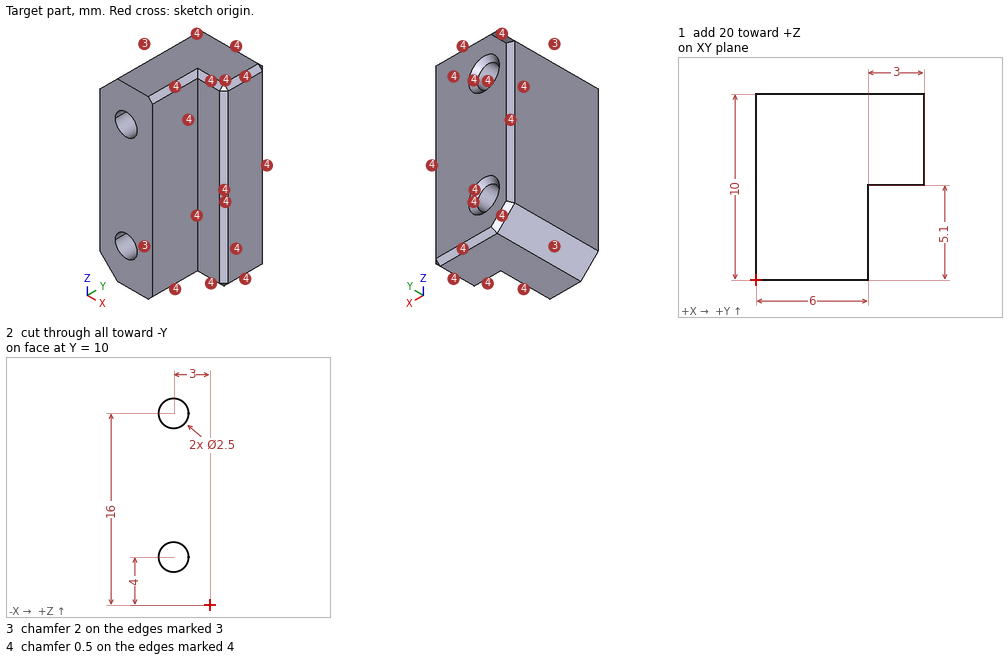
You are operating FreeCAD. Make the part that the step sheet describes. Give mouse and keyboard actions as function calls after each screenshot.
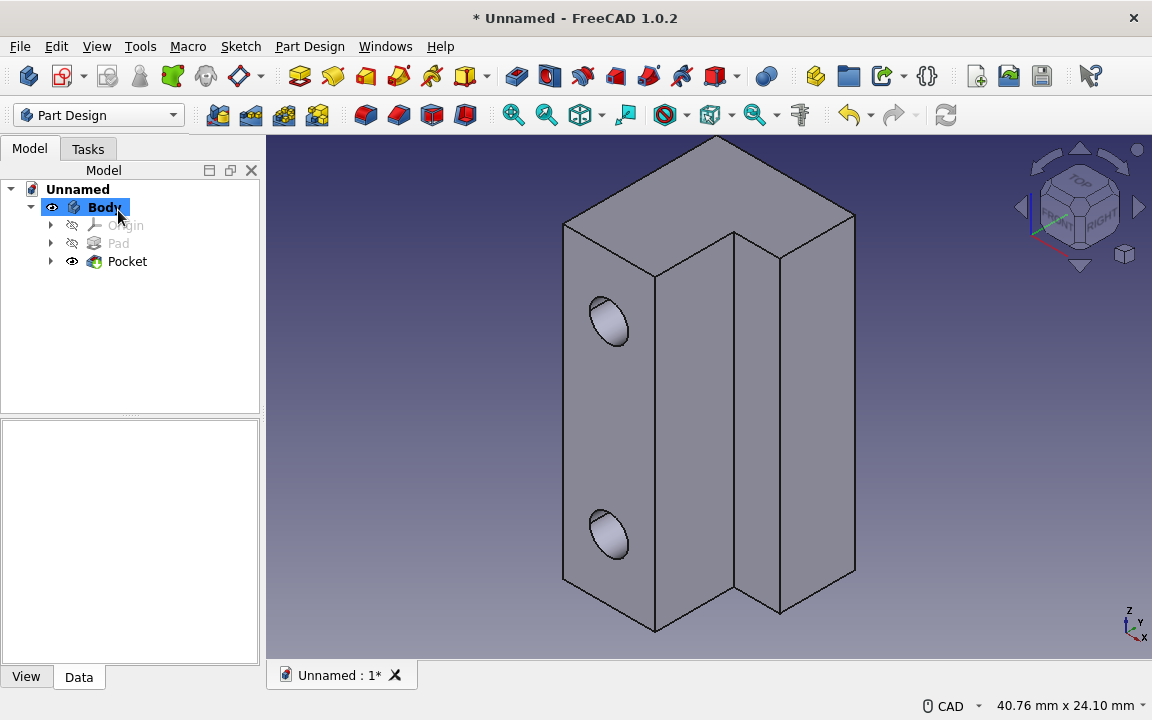
click(514, 116)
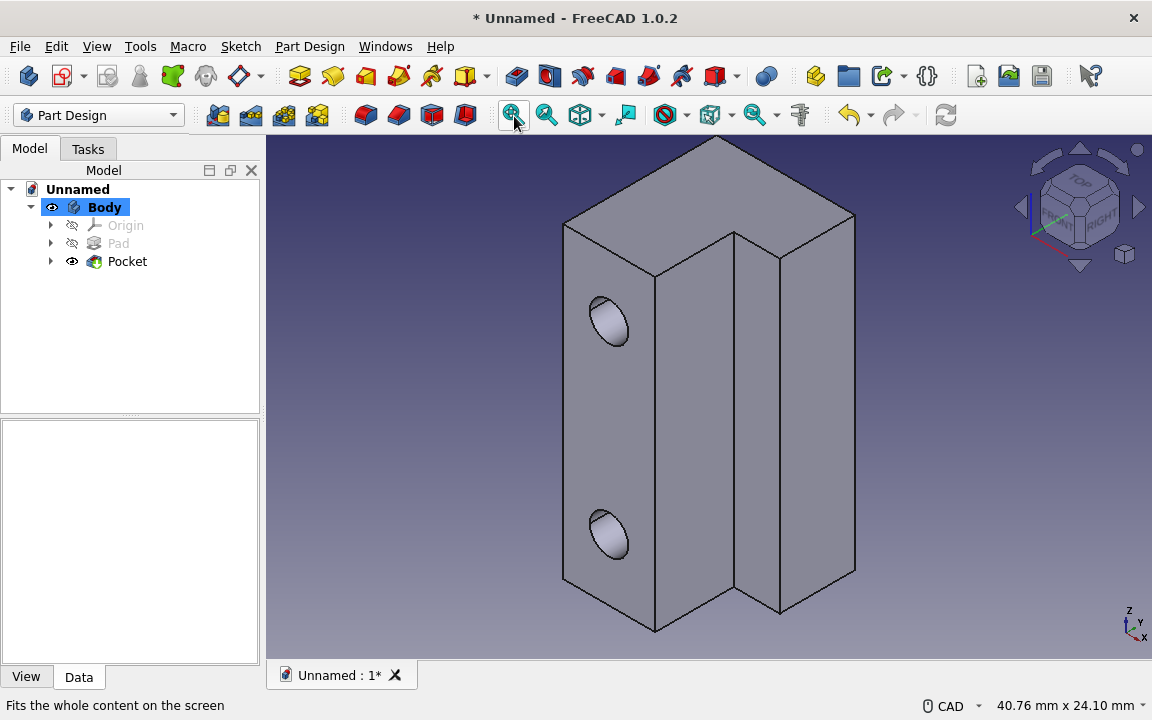
key(2)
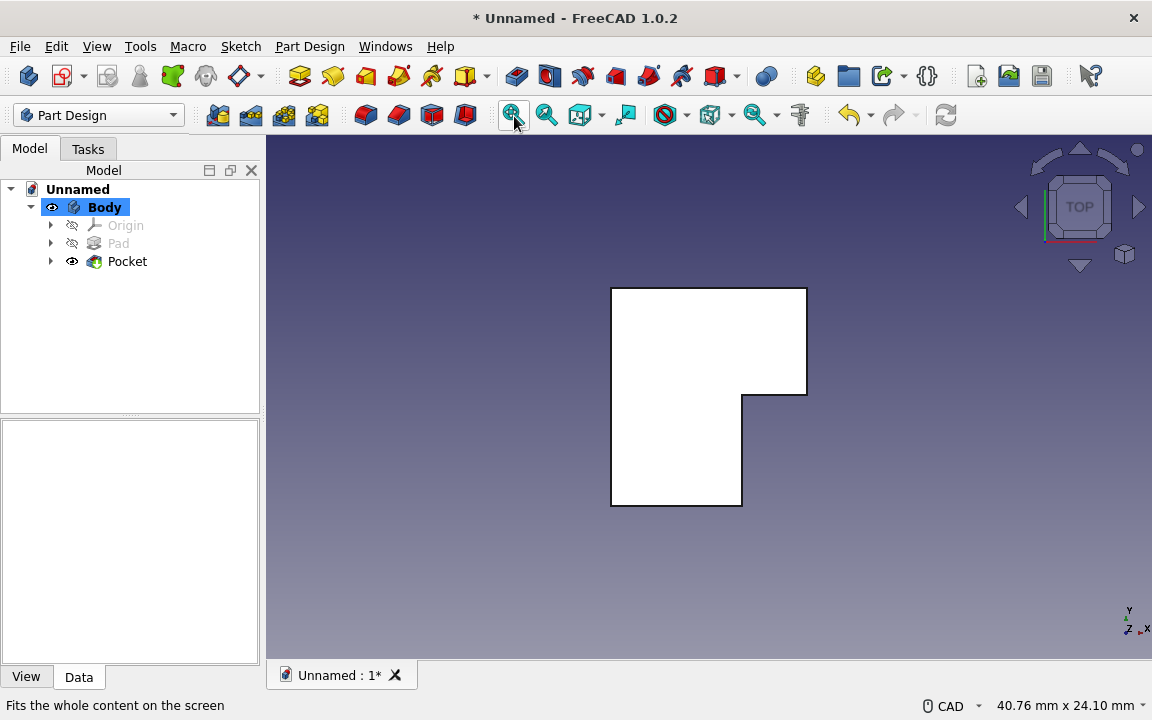
click(514, 116)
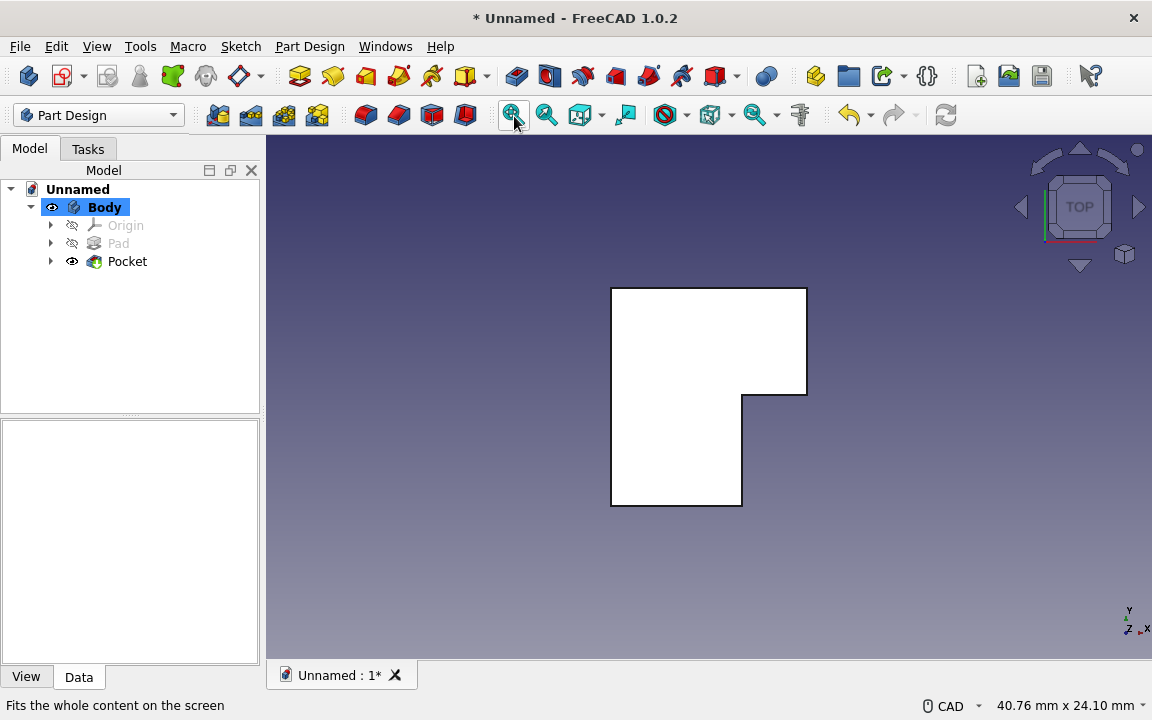
click(611, 396)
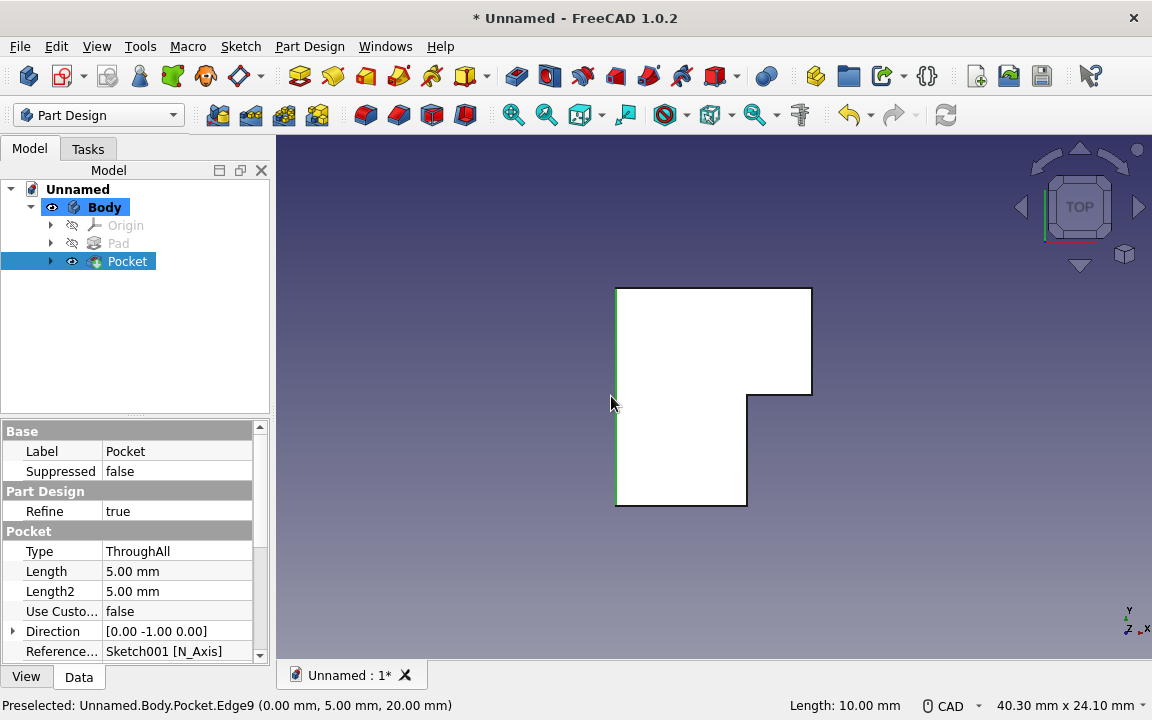
key(1)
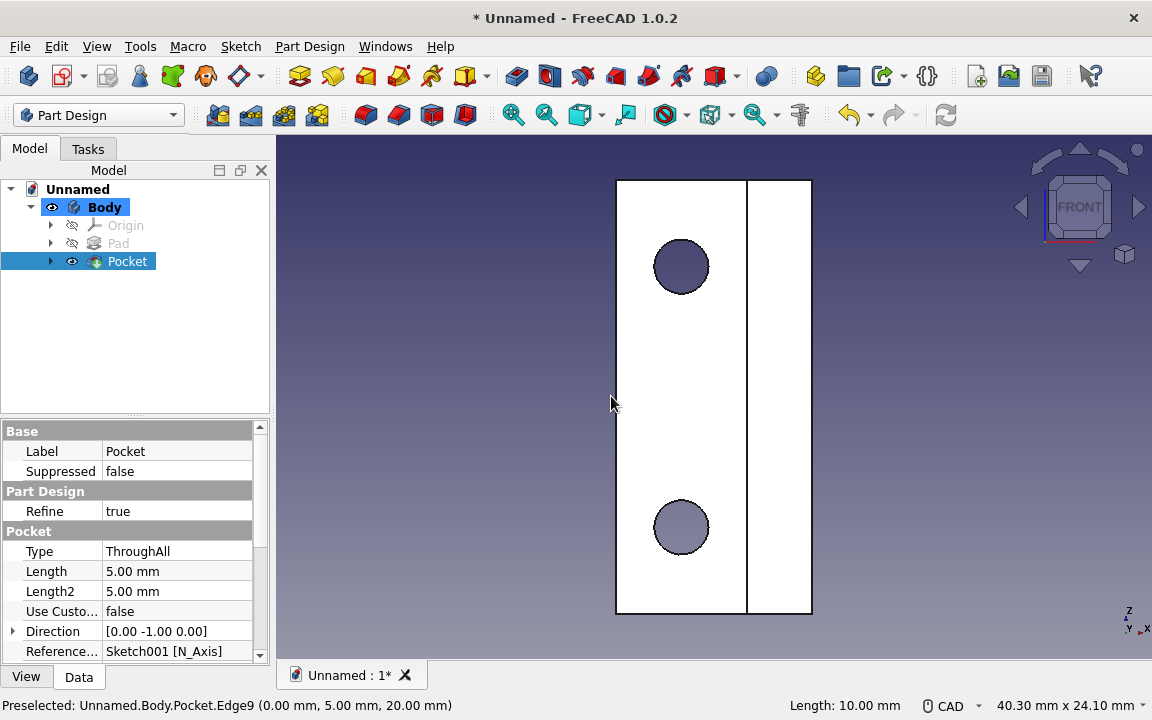
key(3)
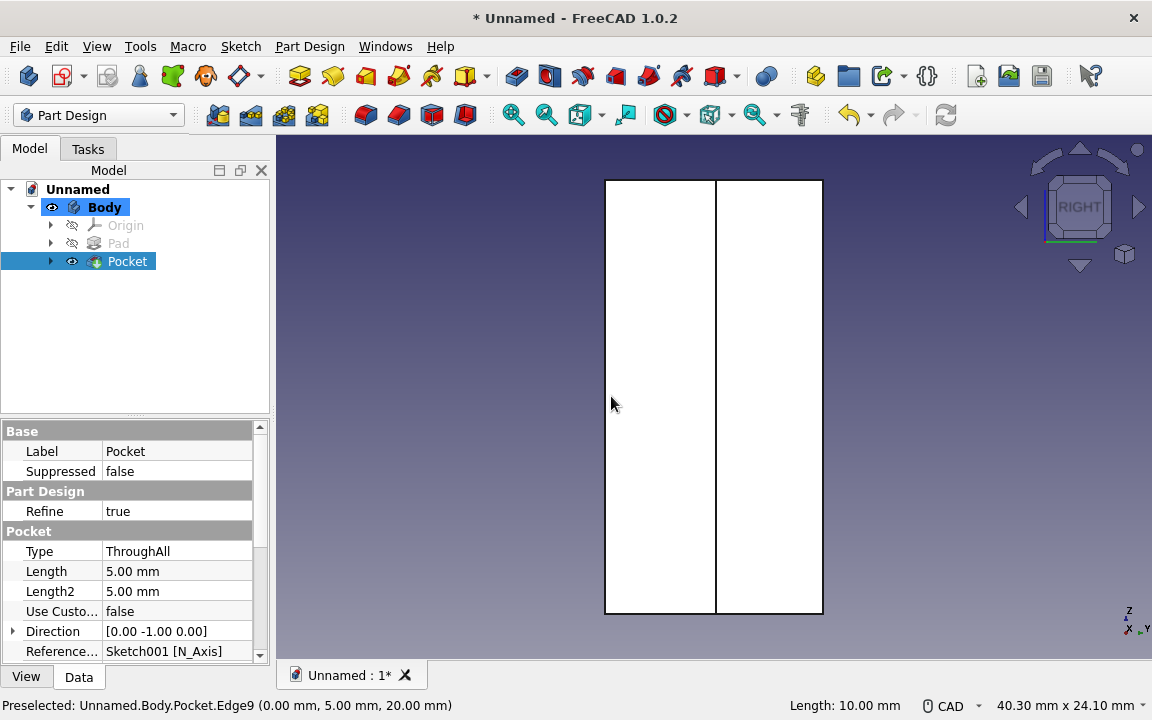
key(5)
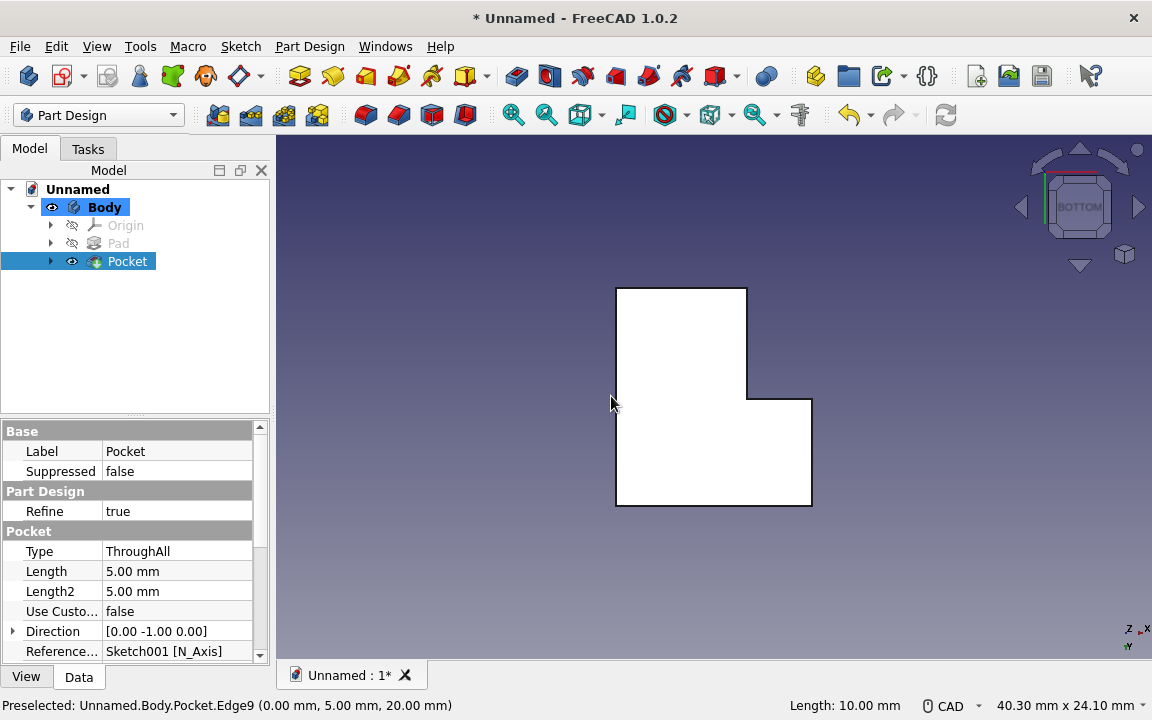
click(514, 116)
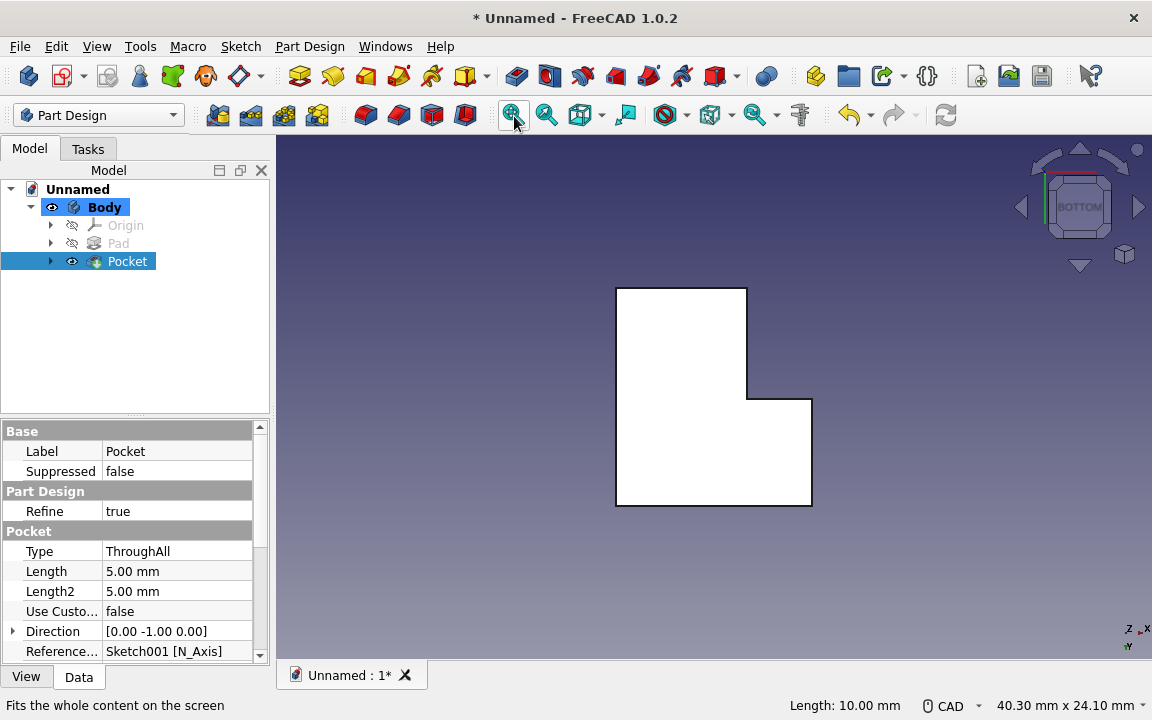
click(616, 396, ctrl)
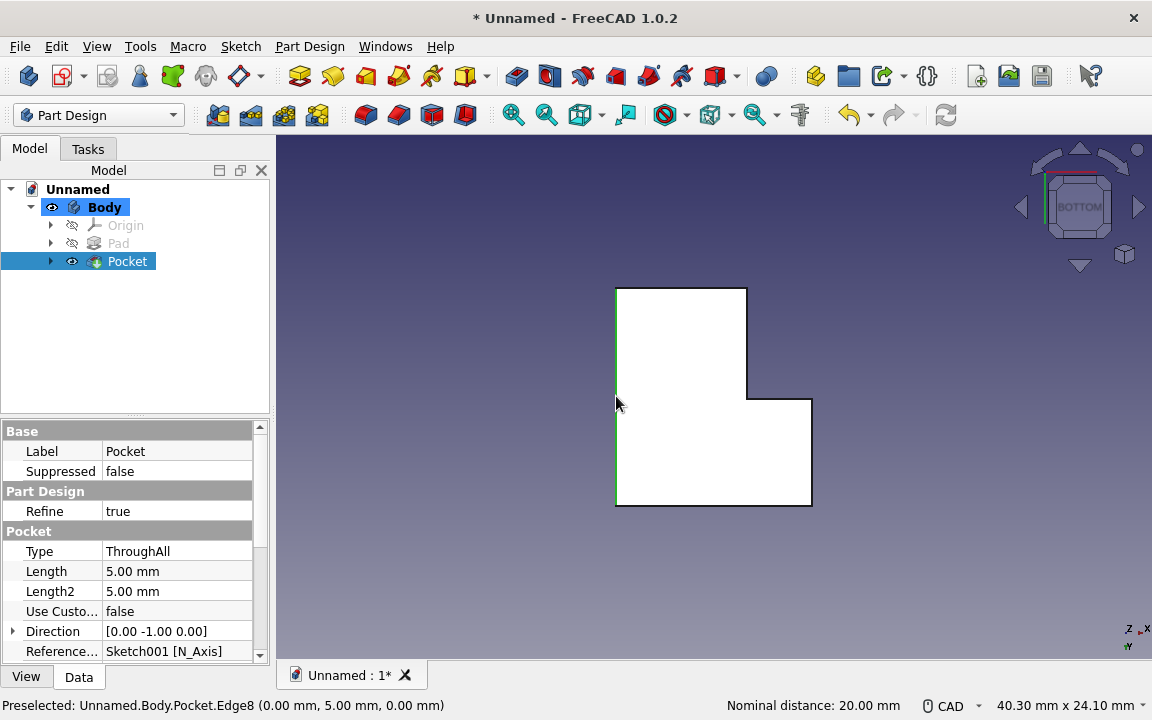
click(399, 116)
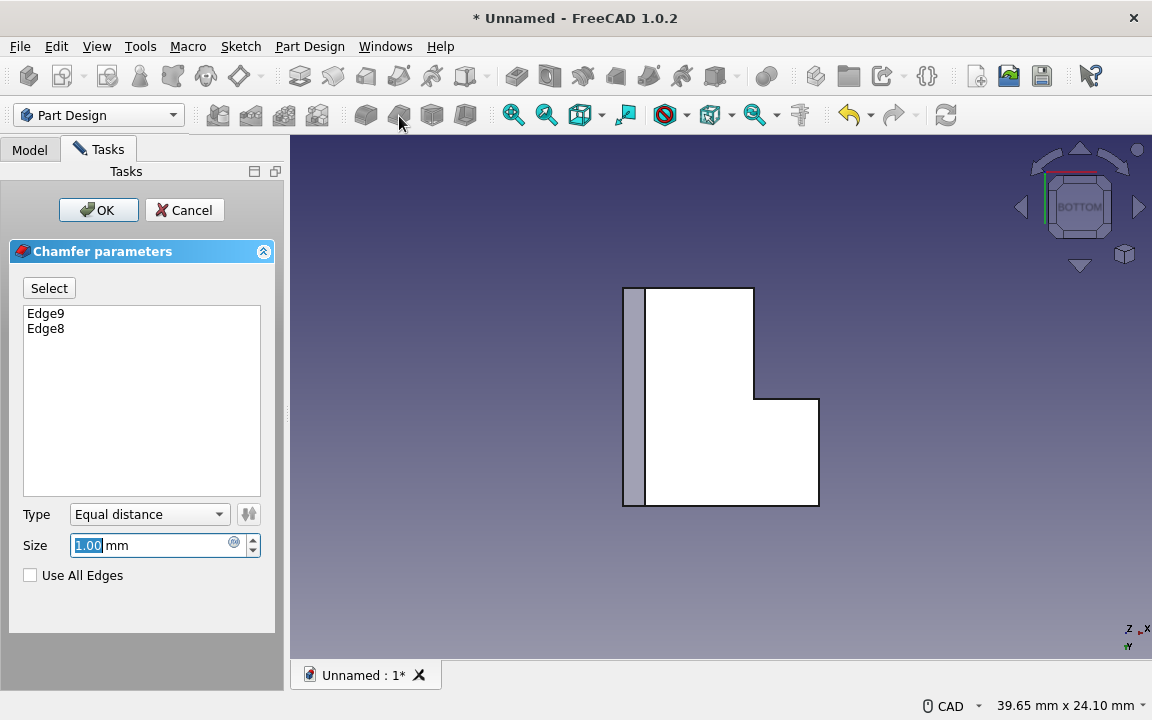
text(2)
key(Tab)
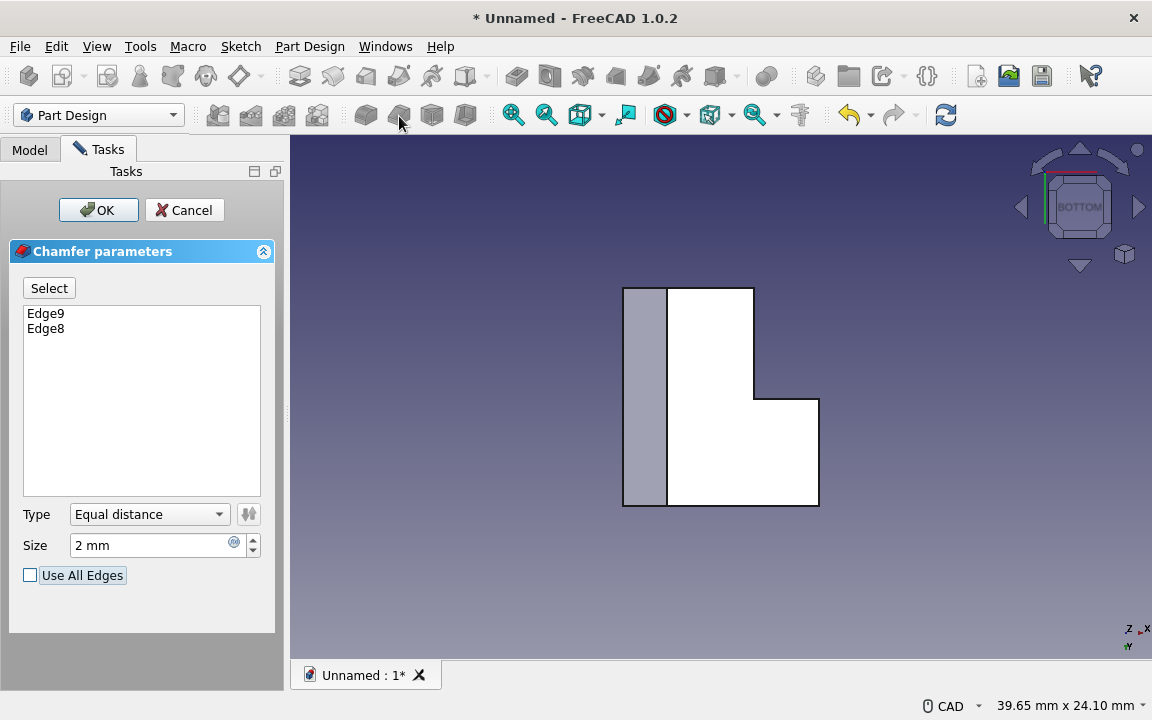
click(99, 210)